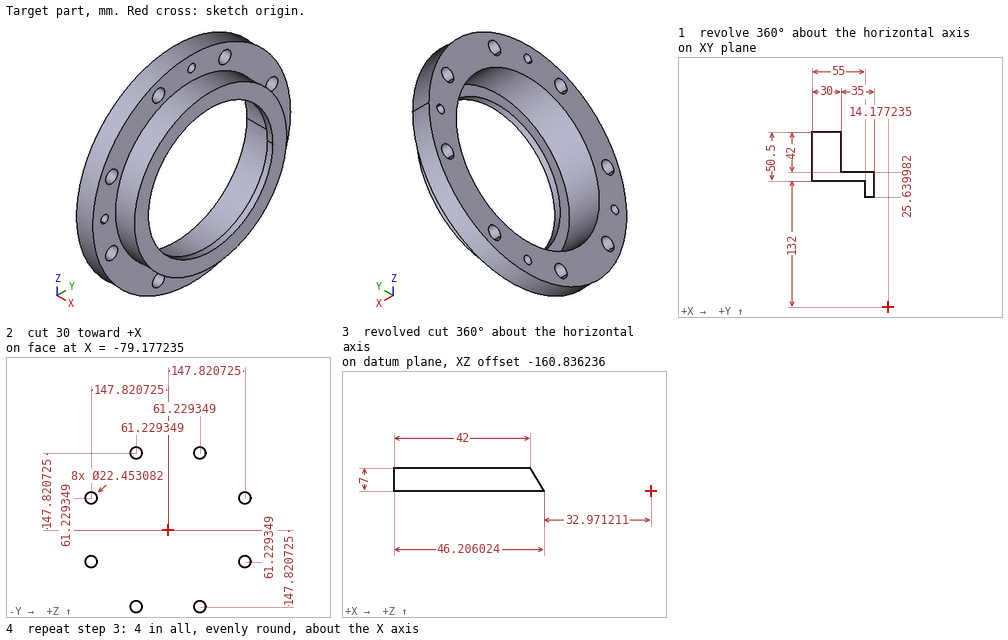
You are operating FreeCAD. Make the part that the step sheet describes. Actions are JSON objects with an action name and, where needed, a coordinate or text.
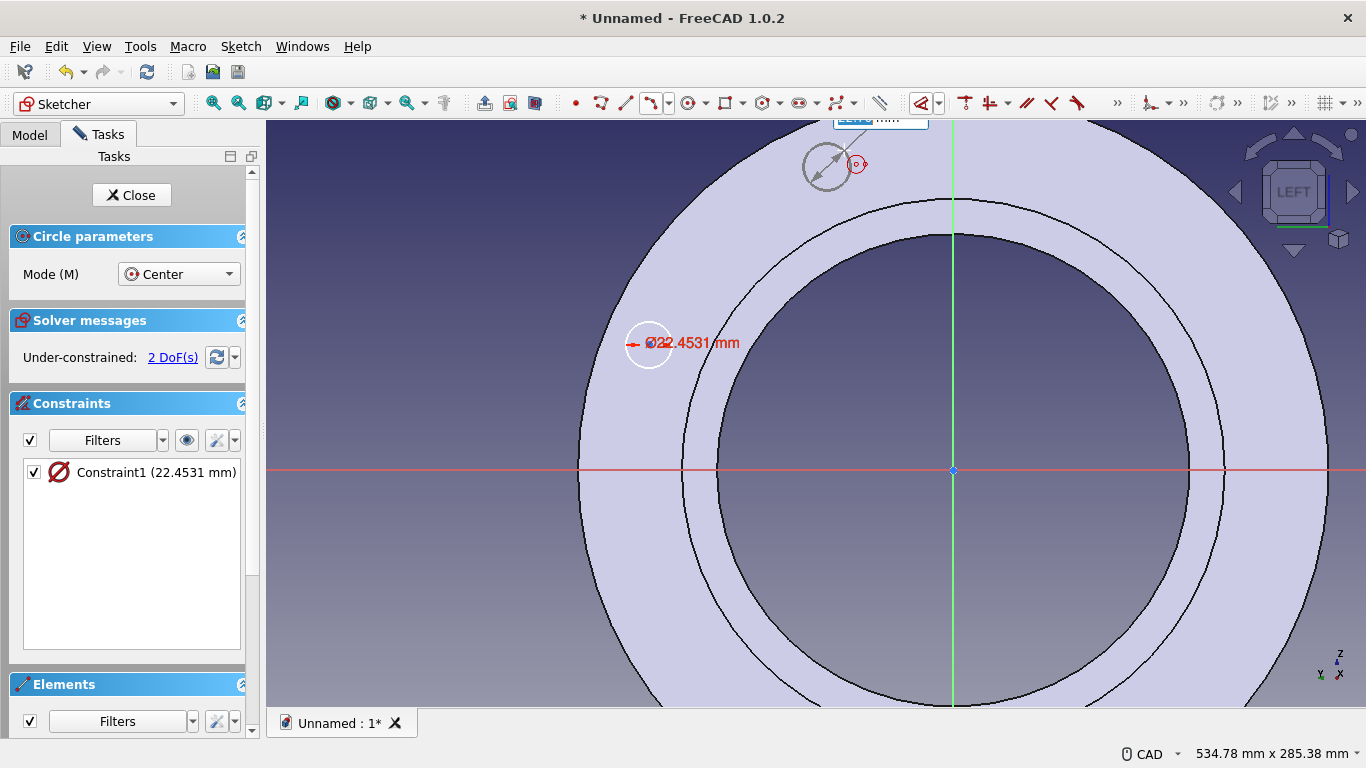
{"action": "type", "text": "22.453082"}
{"action": "key", "text": "Return"}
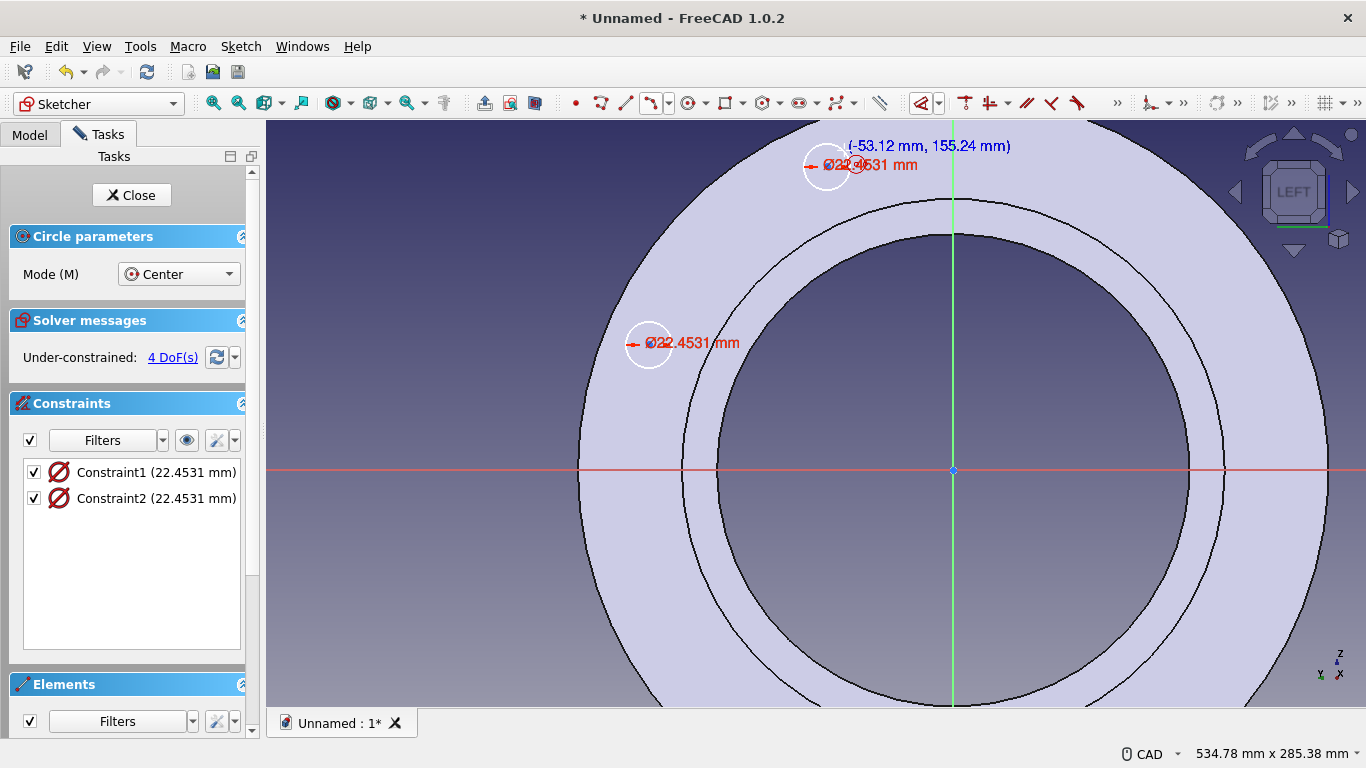
{"action": "left_click", "coordinate": [1079, 166]}
{"action": "mouse_move", "coordinate": [1096, 150]}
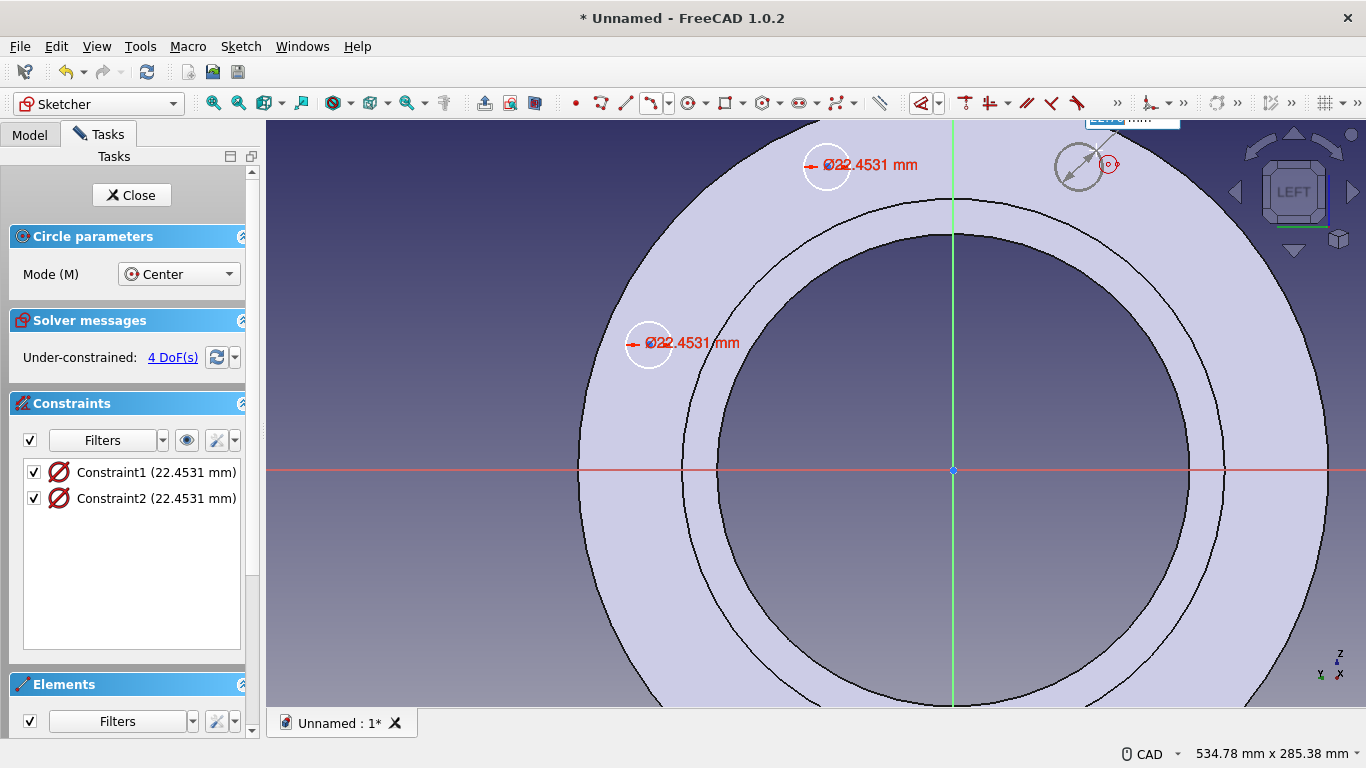
{"action": "type", "text": "22.453082"}
{"action": "key", "text": "Return"}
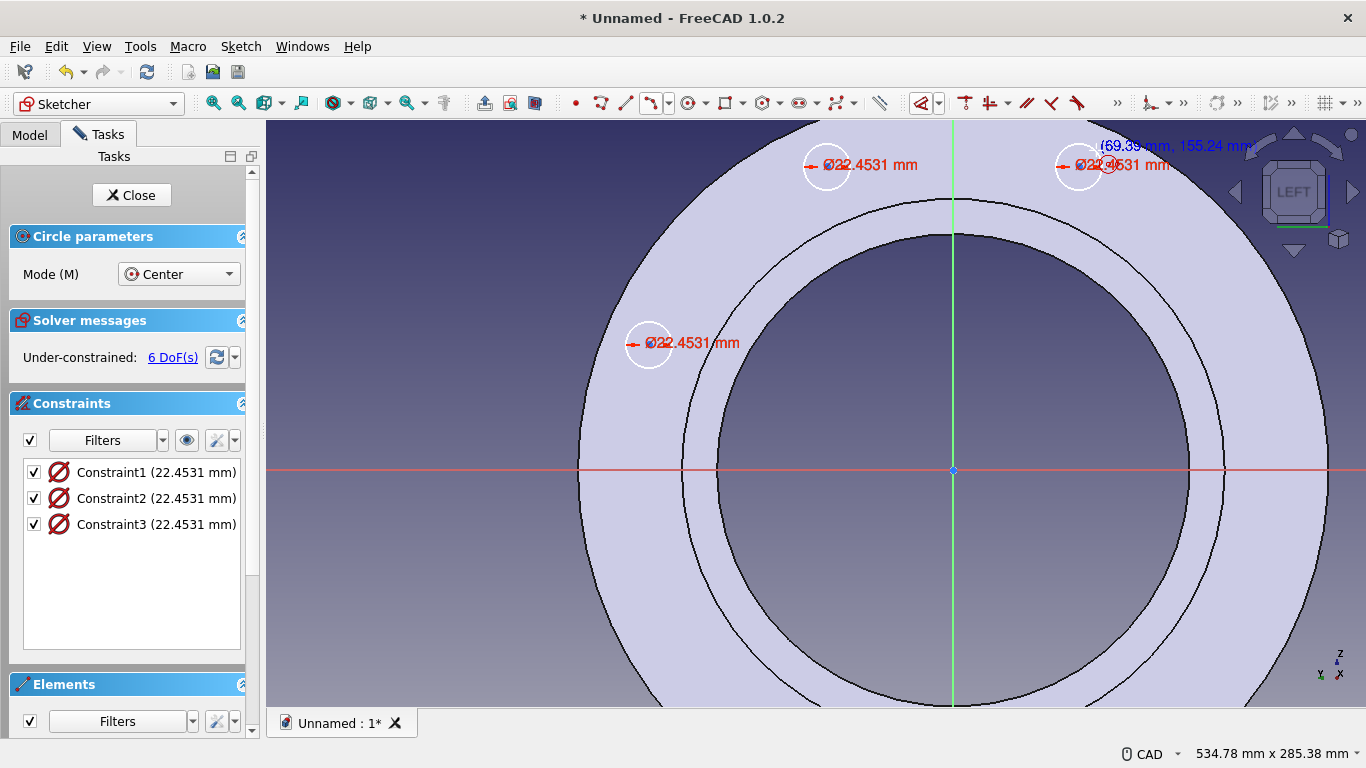
{"action": "scroll", "coordinate": [497, 344], "scroll_direction": "down", "scroll_amount": 3}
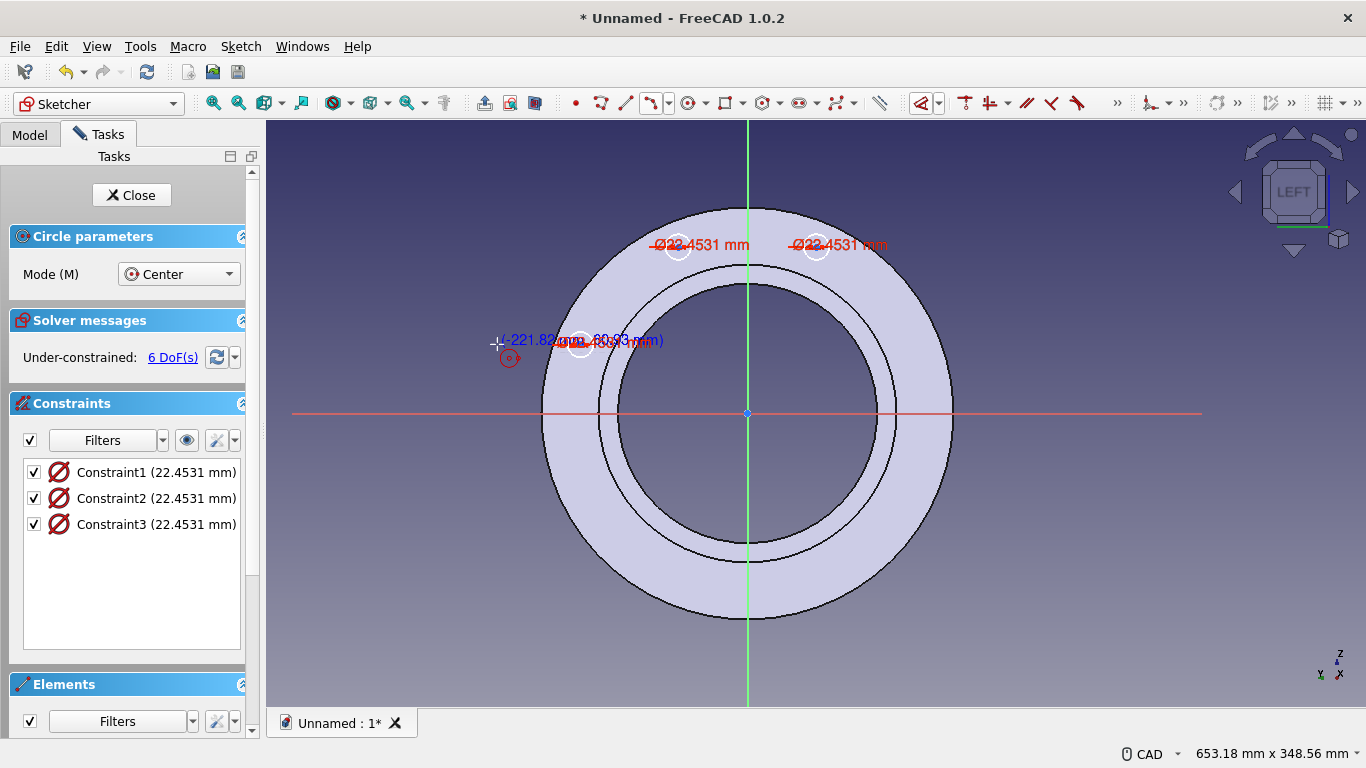
{"action": "scroll", "coordinate": [914, 344], "scroll_direction": "up", "scroll_amount": 3}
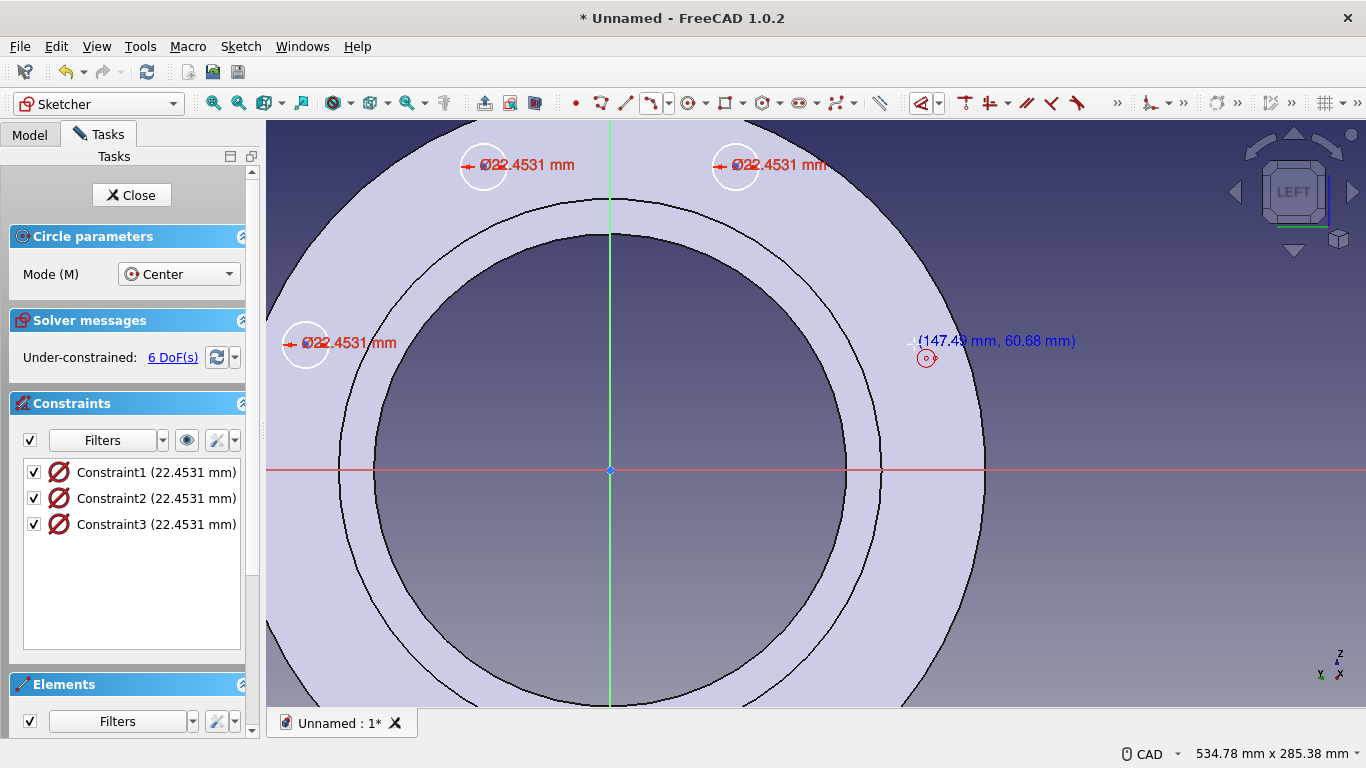
{"action": "left_click", "coordinate": [914, 344]}
{"action": "mouse_move", "coordinate": [931, 328]}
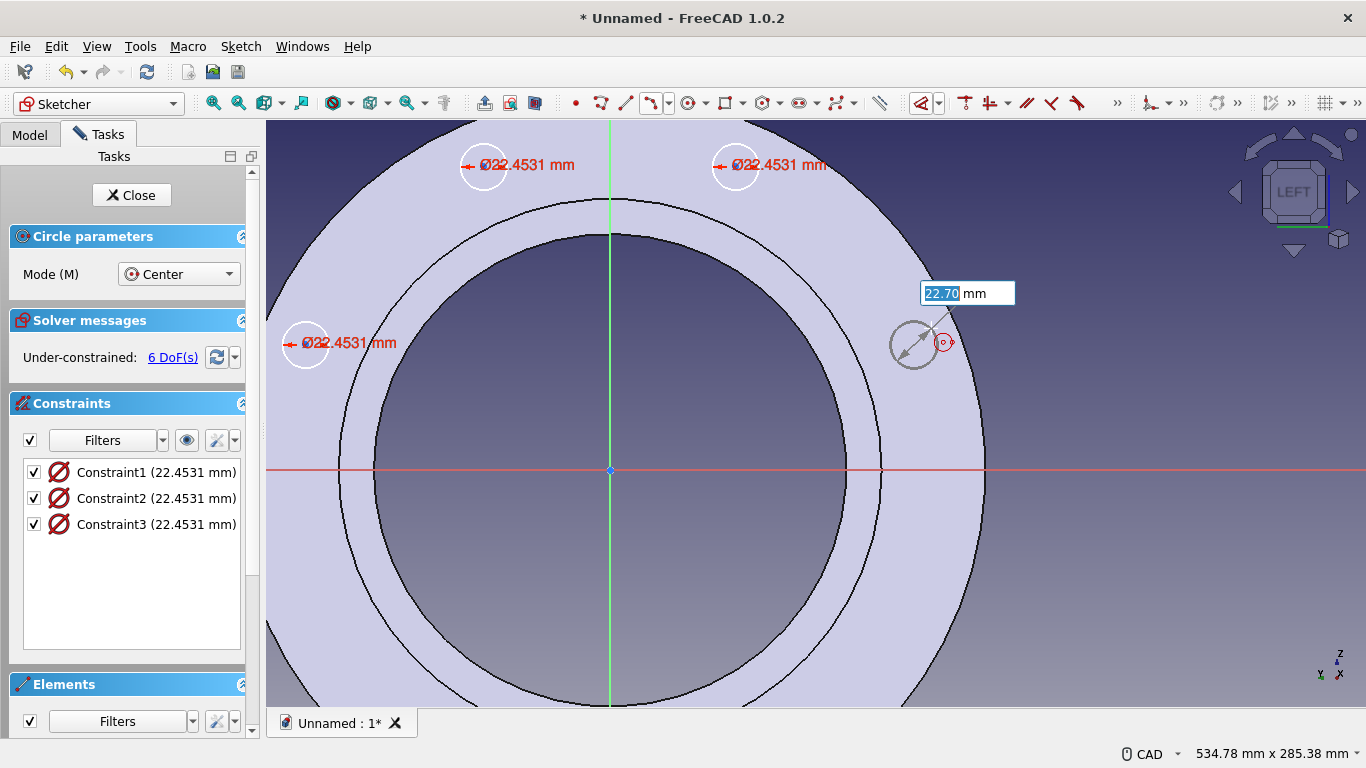
{"action": "type", "text": "22.453082"}
{"action": "key", "text": "Return"}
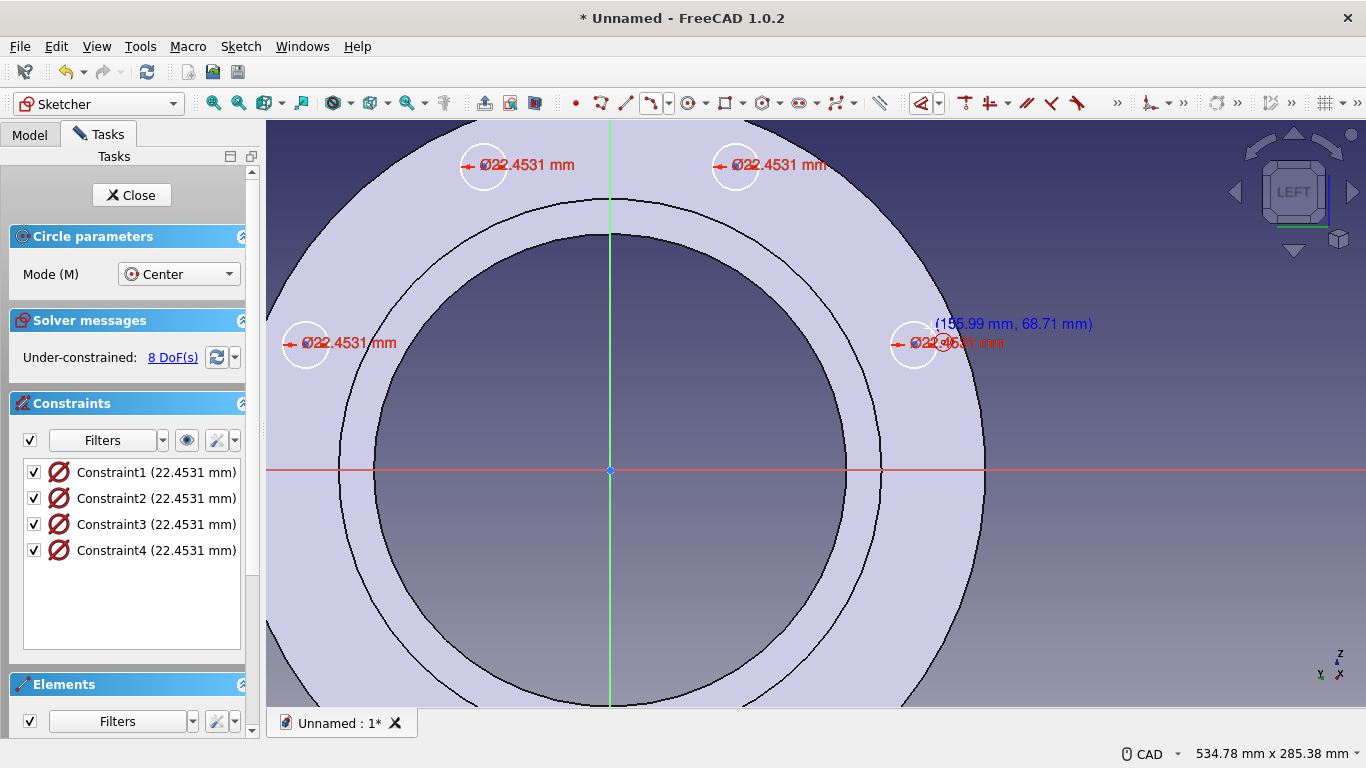
{"action": "left_click", "coordinate": [914, 596]}
{"action": "mouse_move", "coordinate": [931, 580]}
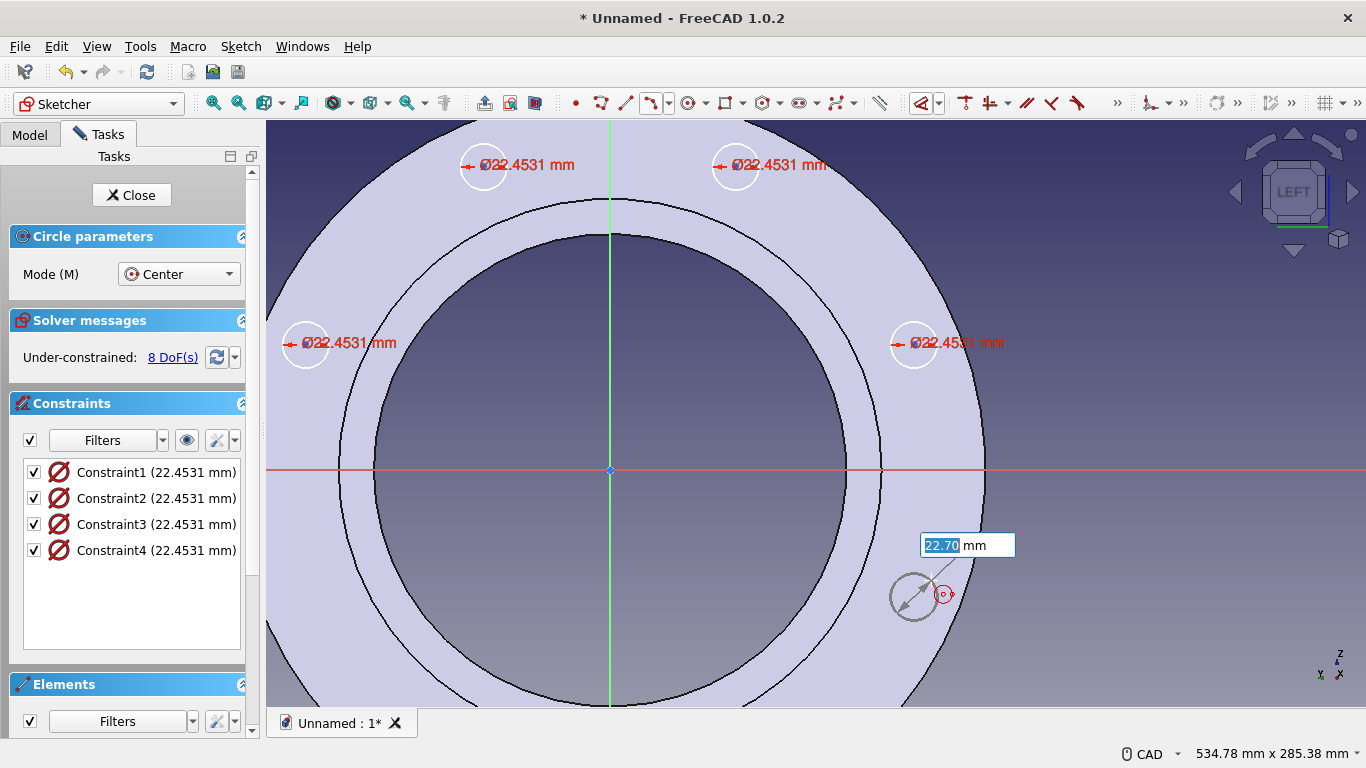
{"action": "type", "text": "22.453082"}
{"action": "key", "text": "Return"}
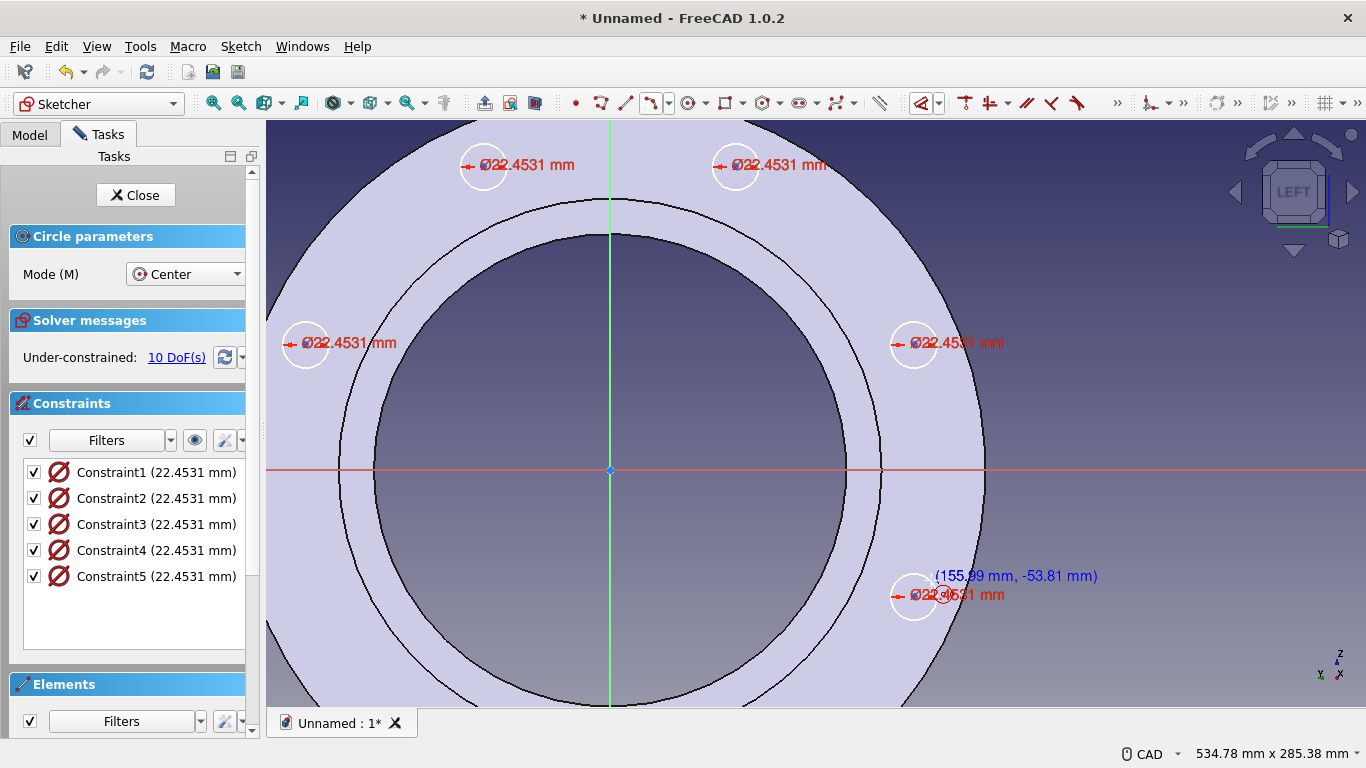
{"action": "scroll", "coordinate": [915, 344], "scroll_direction": "down", "scroll_amount": 3}